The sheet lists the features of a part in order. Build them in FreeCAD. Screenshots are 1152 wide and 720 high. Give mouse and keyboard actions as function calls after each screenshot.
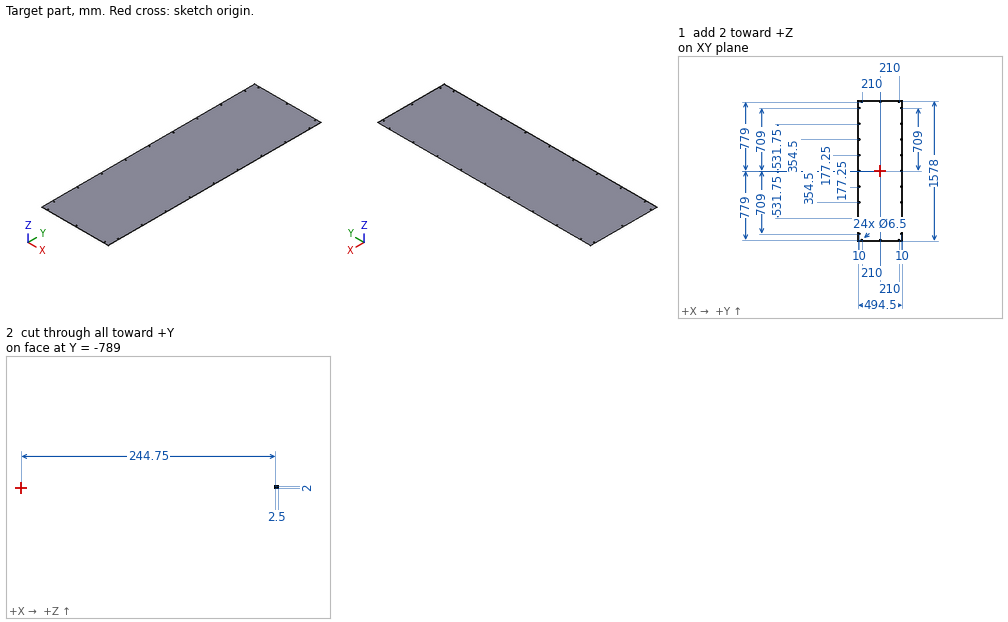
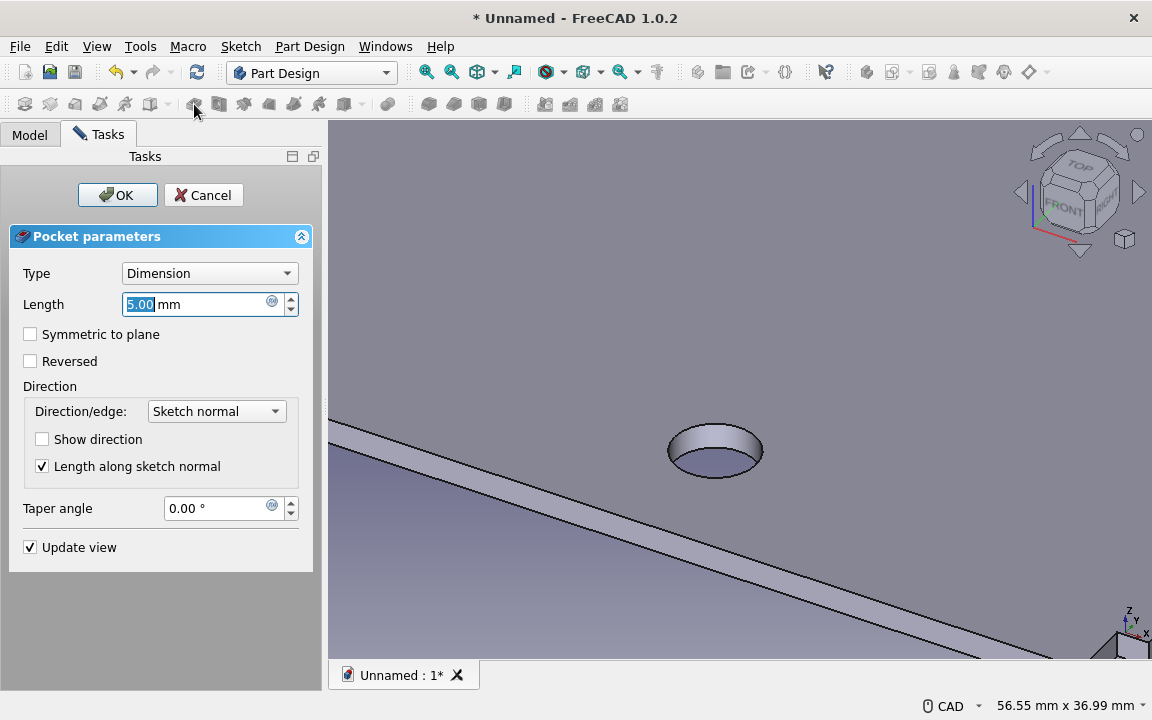
click(210, 274)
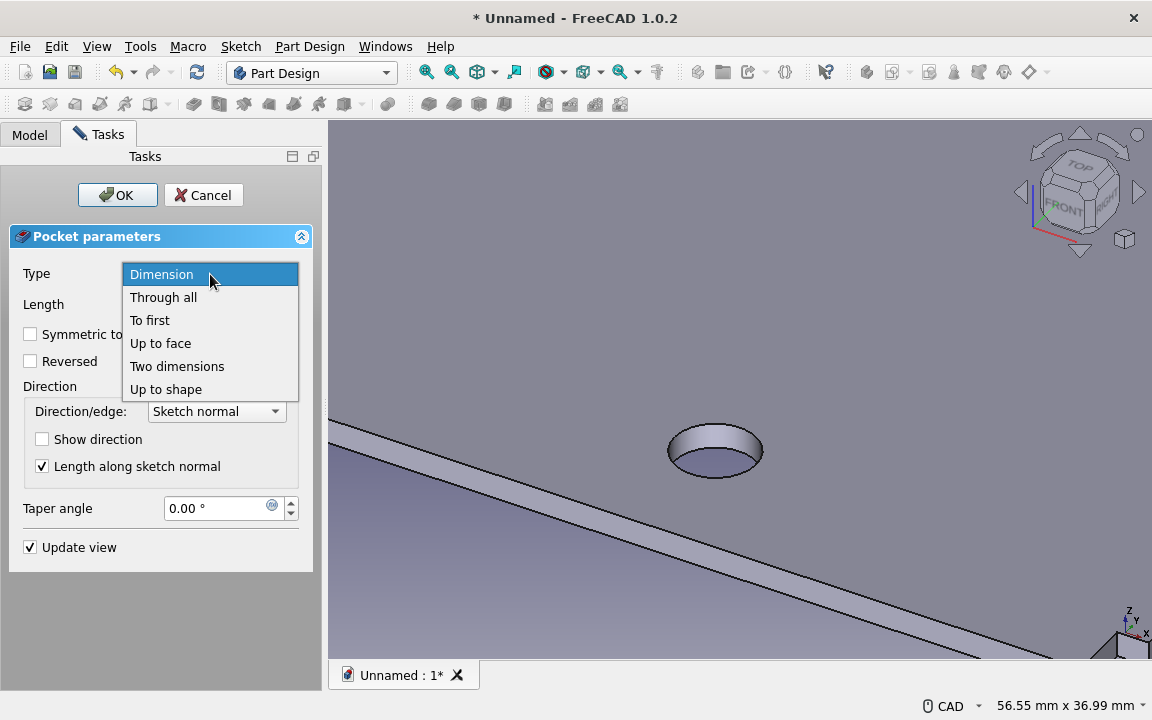
click(208, 298)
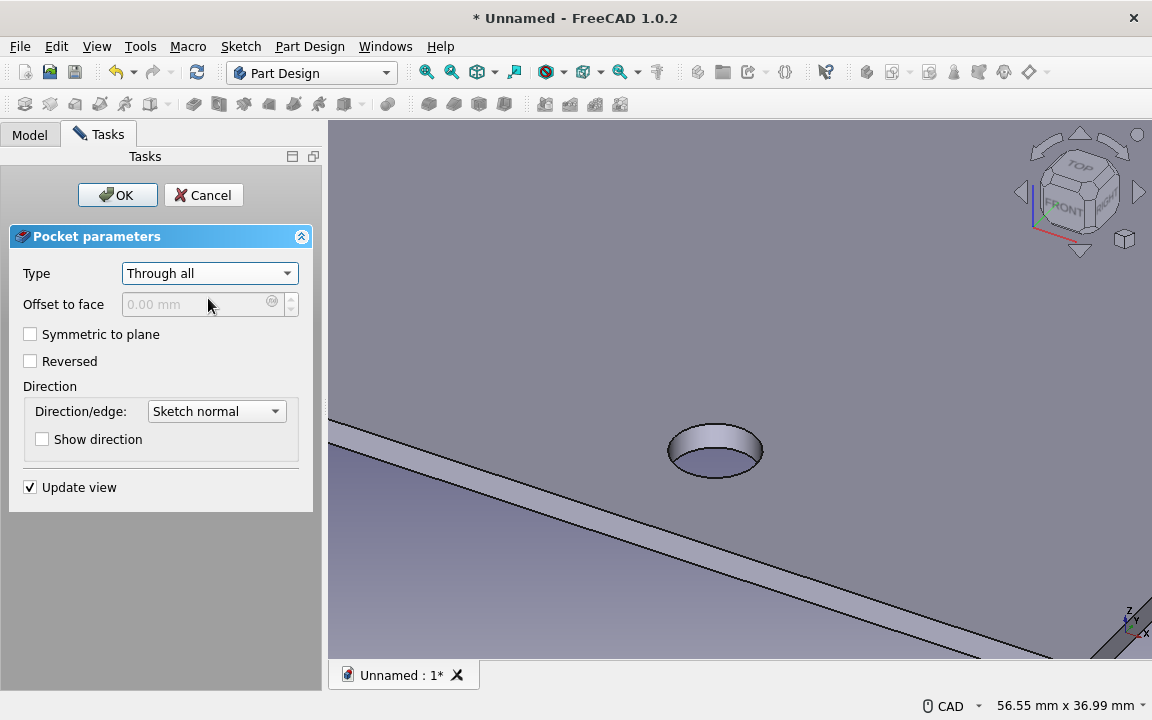
click(118, 195)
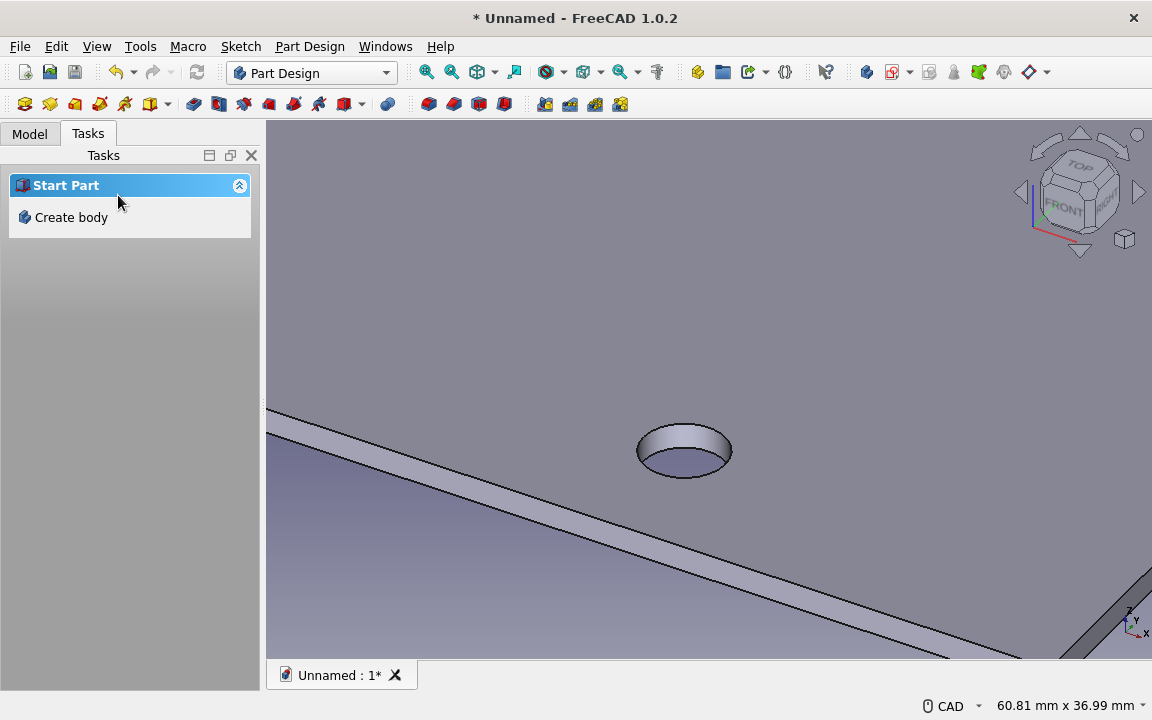
key(0)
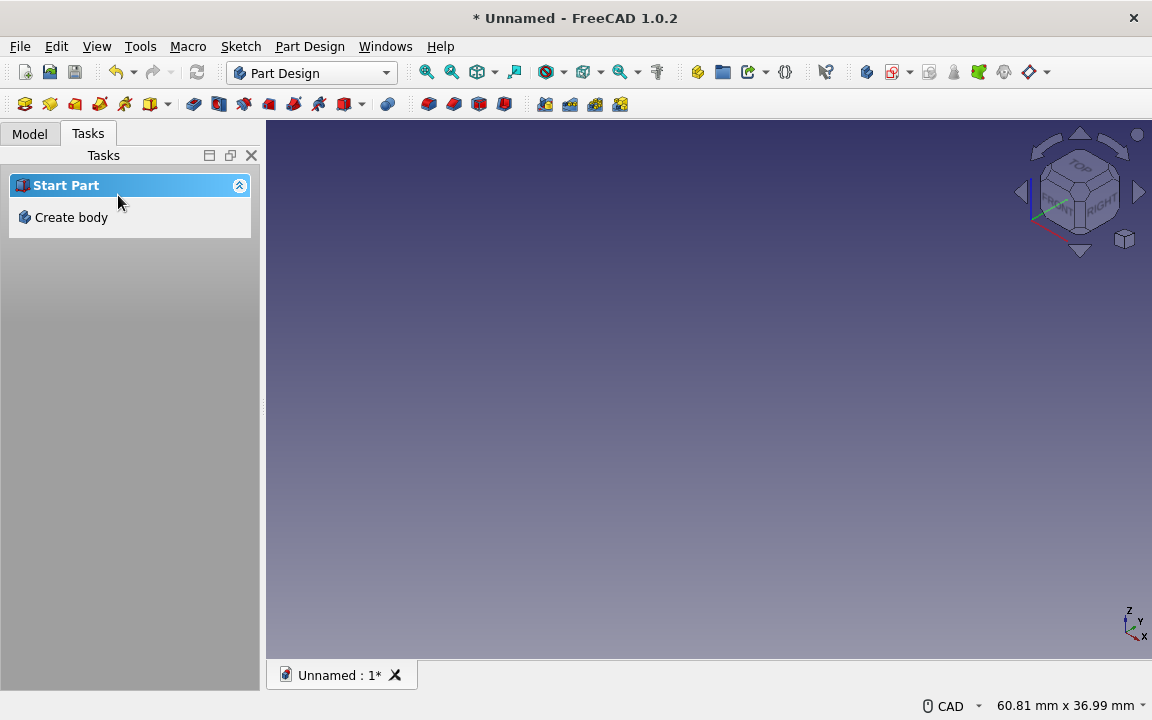
click(427, 72)